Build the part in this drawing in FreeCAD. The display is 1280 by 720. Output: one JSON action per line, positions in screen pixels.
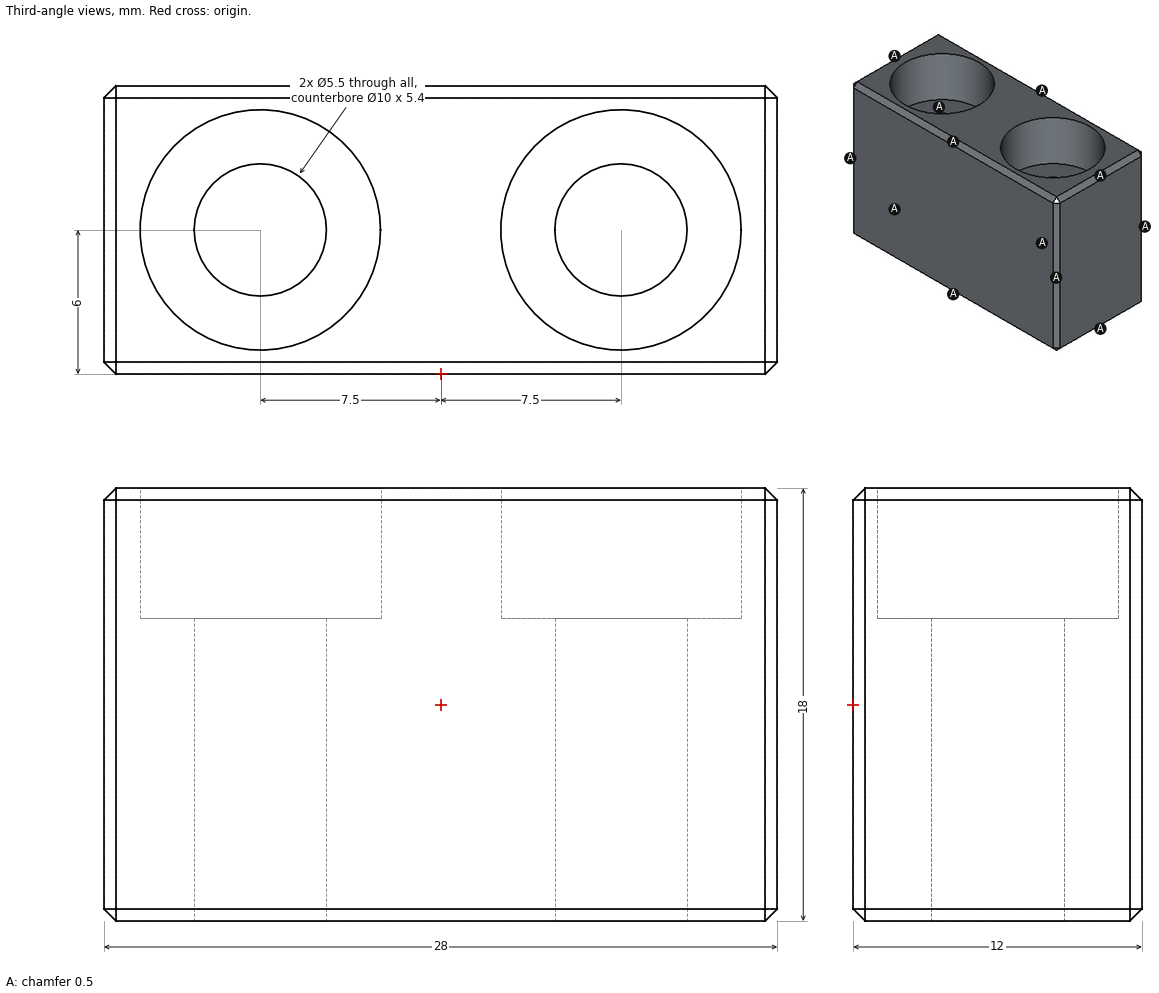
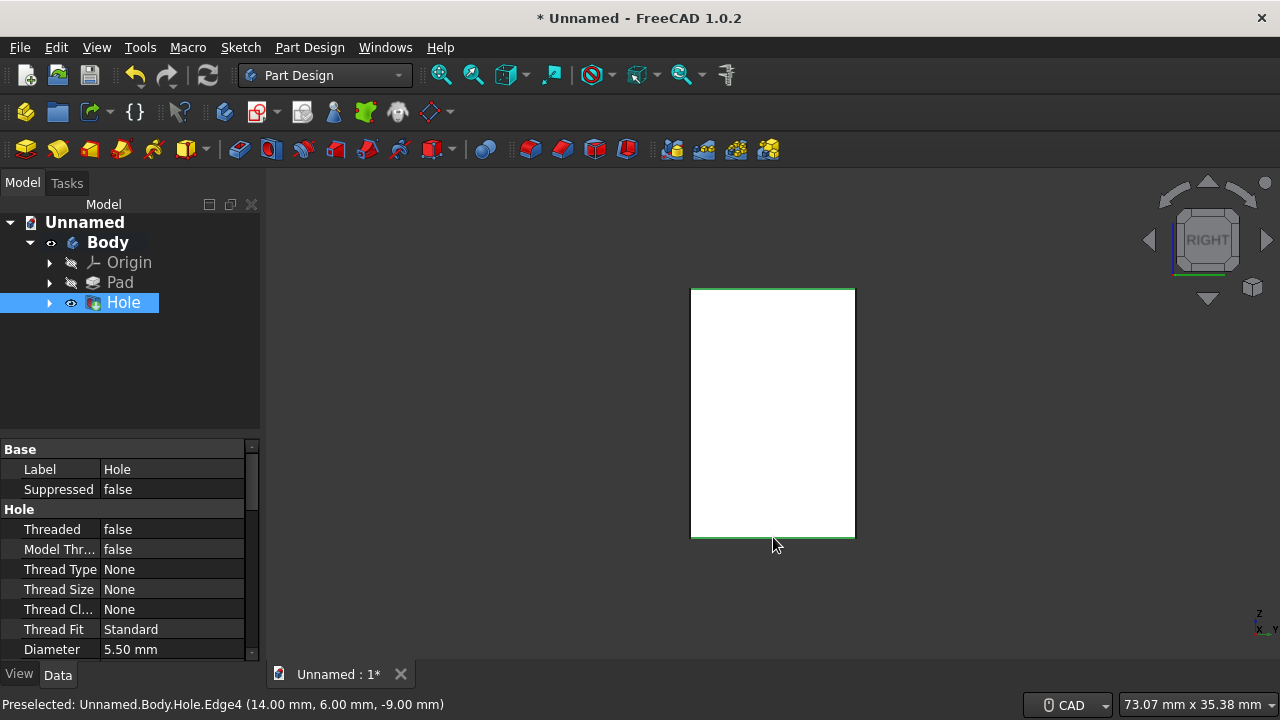
{"action": "key", "text": "5"}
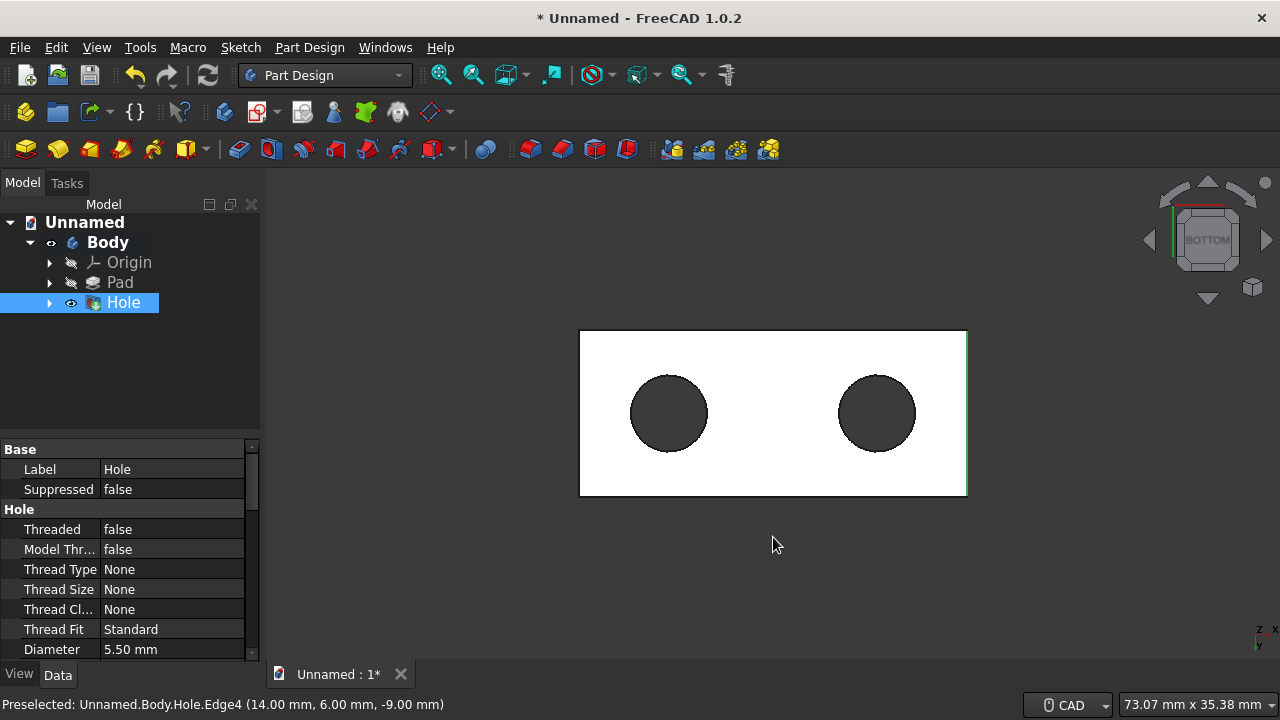
{"action": "left_click", "coordinate": [442, 76]}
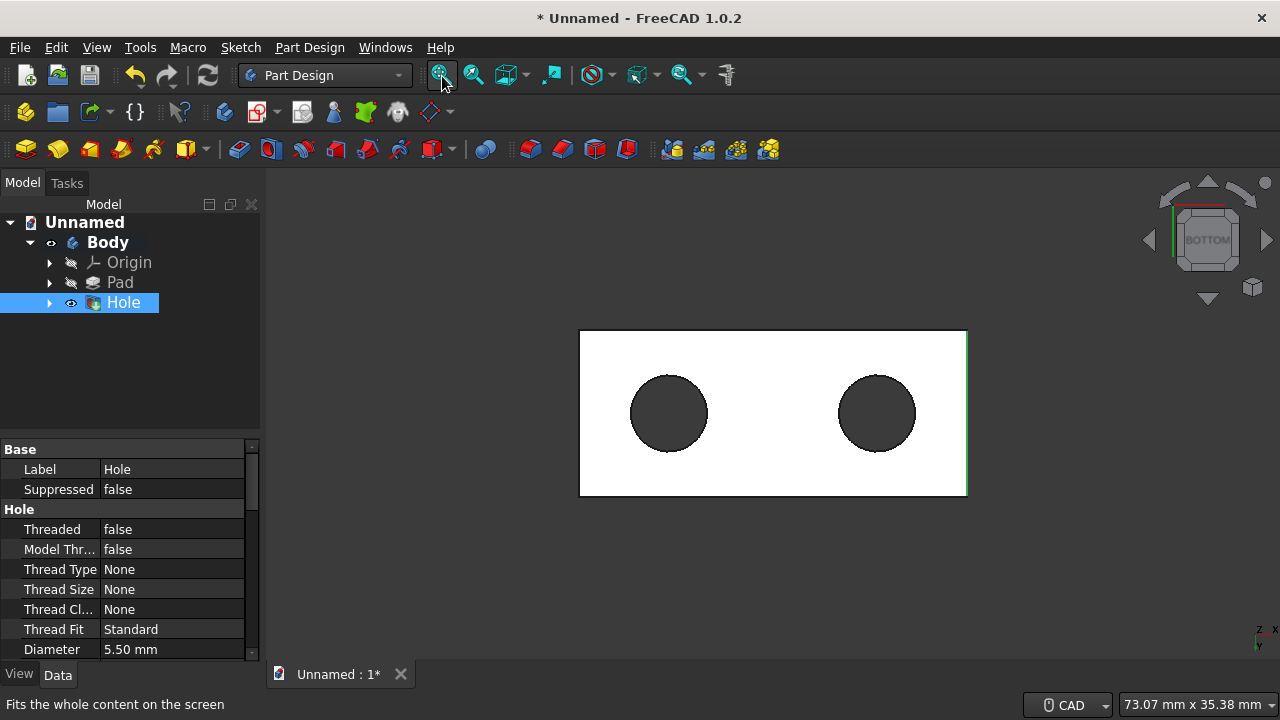
{"action": "left_click", "coordinate": [579, 412], "text": "ctrl"}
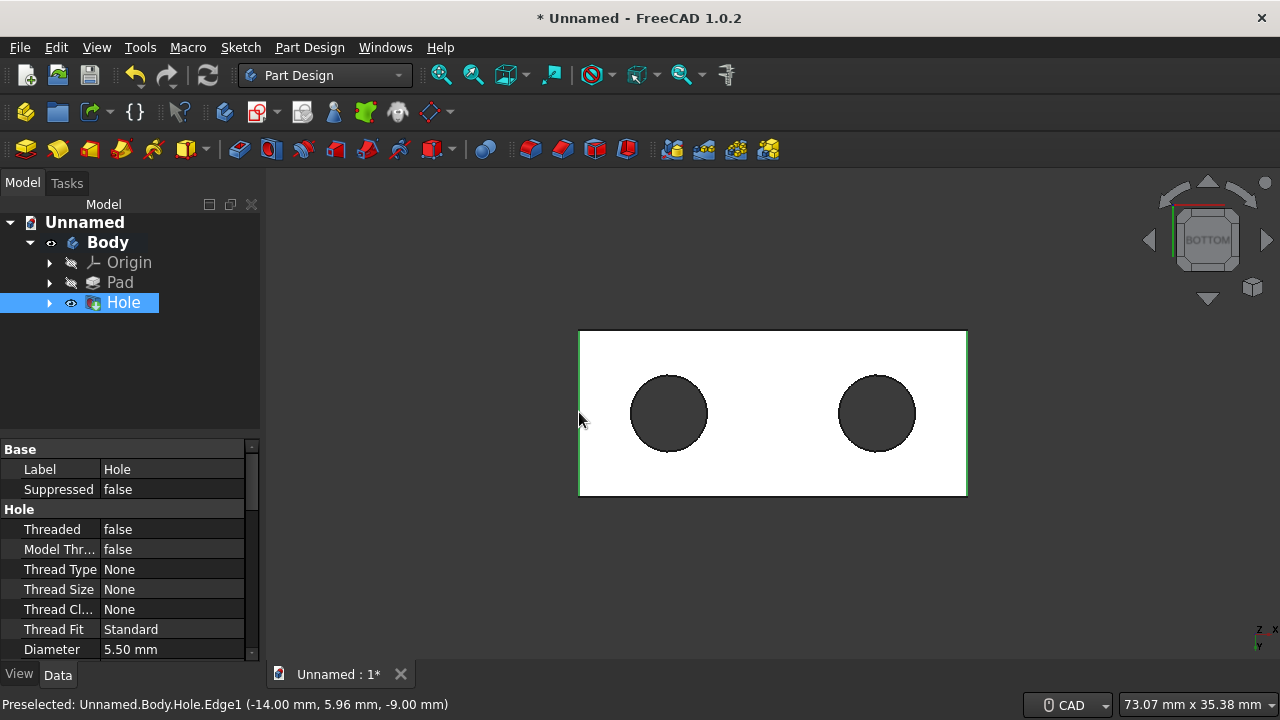
{"action": "key", "text": "4"}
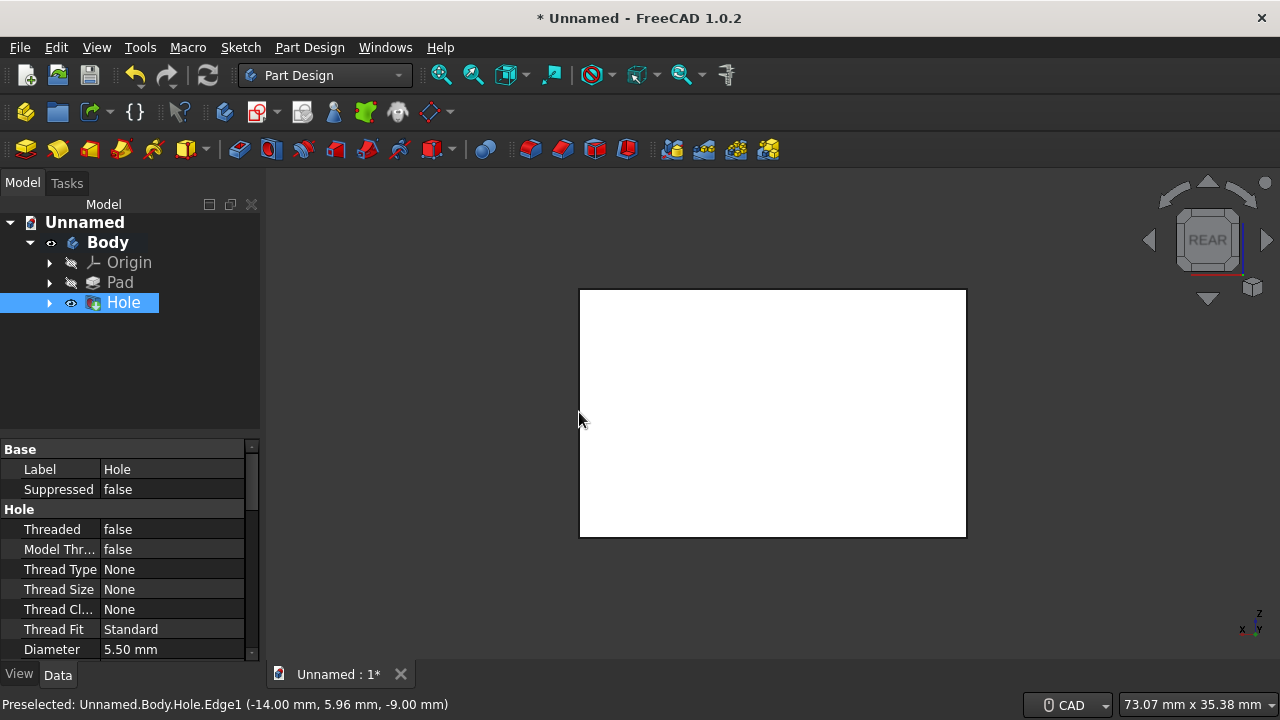
{"action": "left_click", "coordinate": [717, 412], "text": "ctrl"}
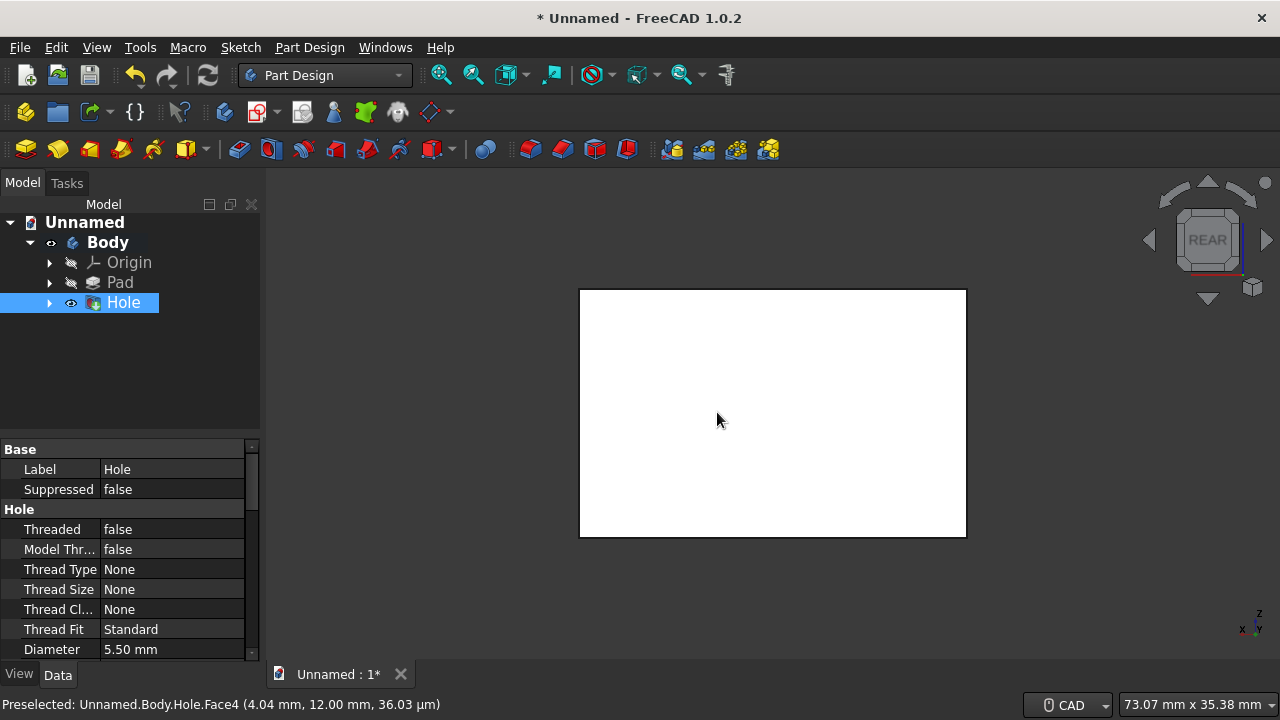
{"action": "left_click", "coordinate": [564, 150]}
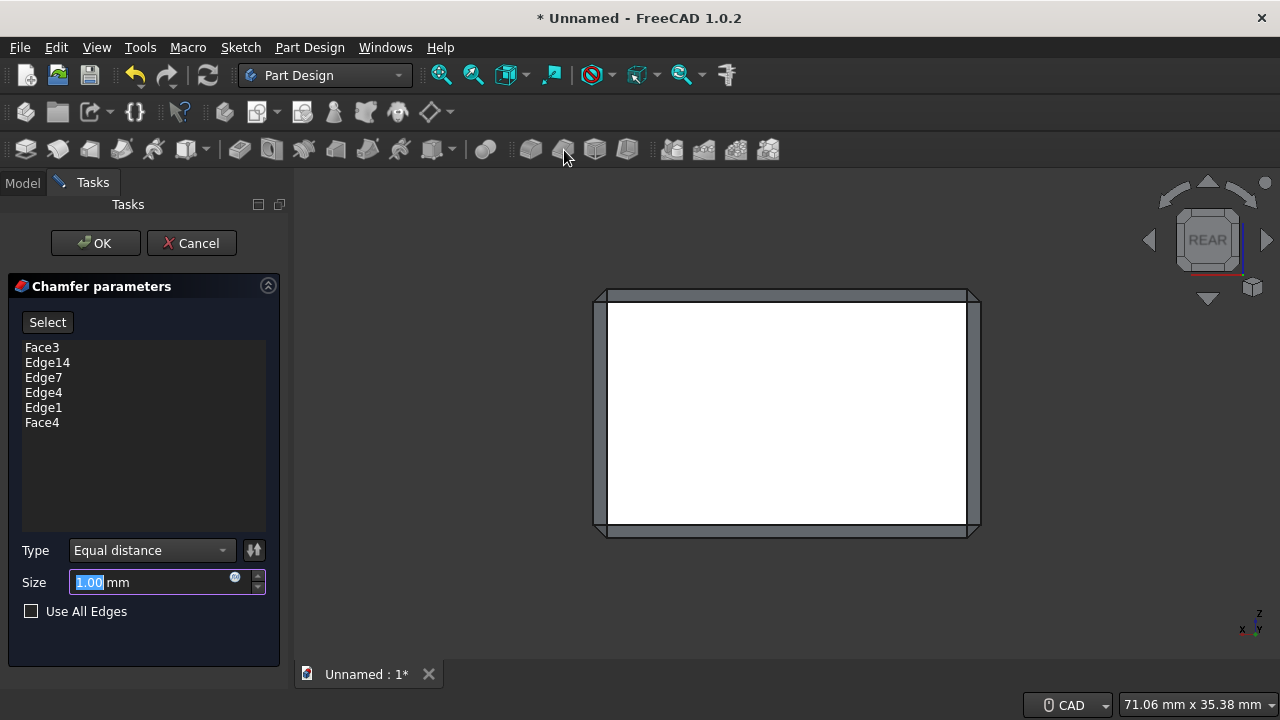
{"action": "type", "text": "0.5"}
{"action": "key", "text": "Tab"}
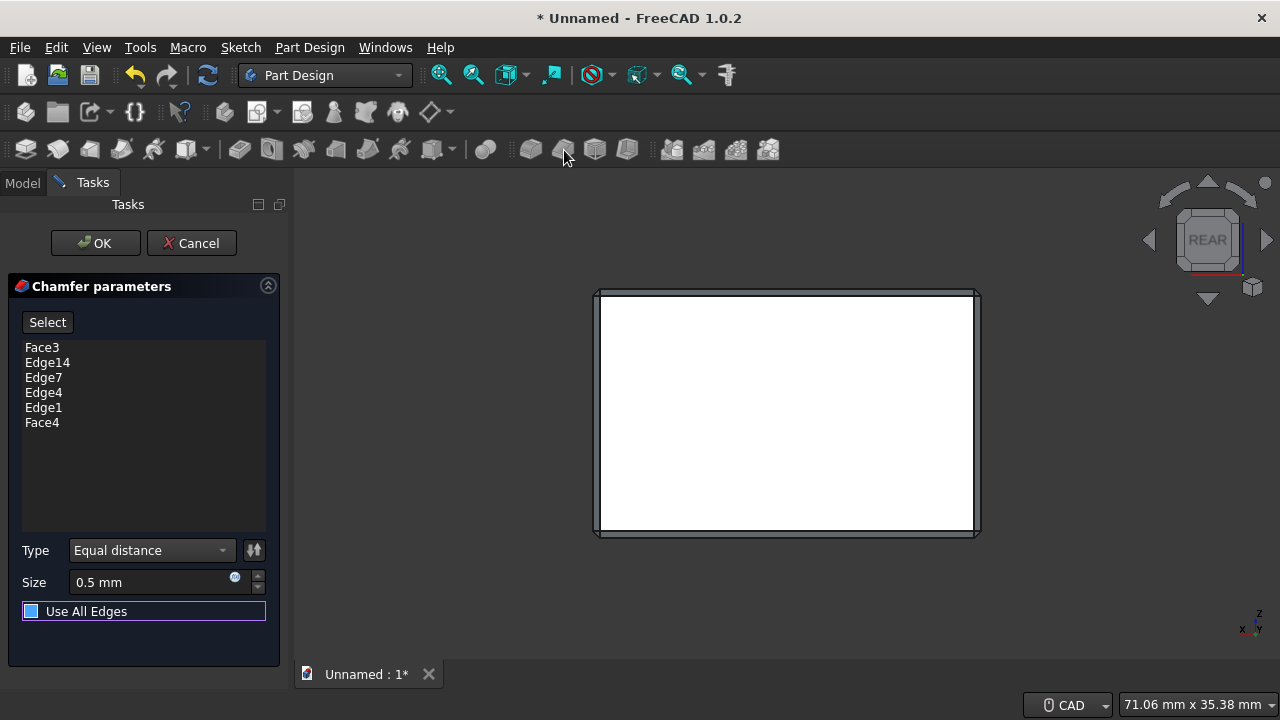
{"action": "left_click", "coordinate": [96, 243]}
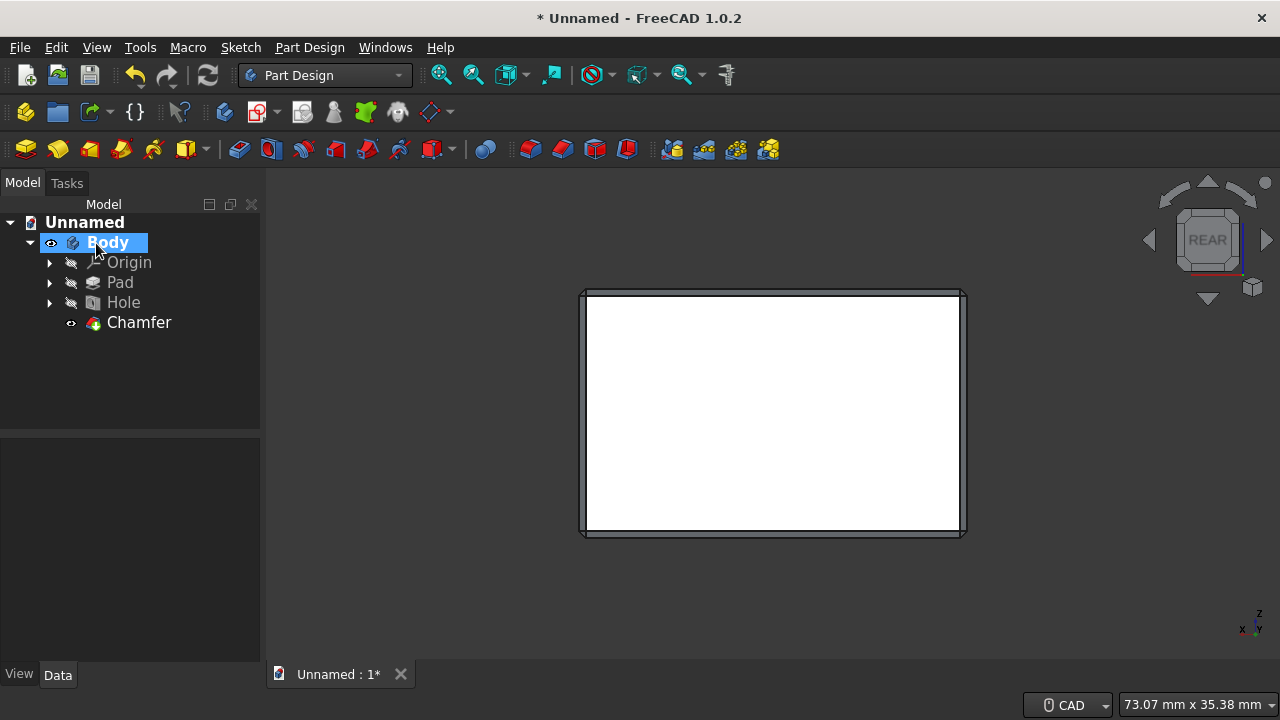
{"action": "key", "text": "0"}